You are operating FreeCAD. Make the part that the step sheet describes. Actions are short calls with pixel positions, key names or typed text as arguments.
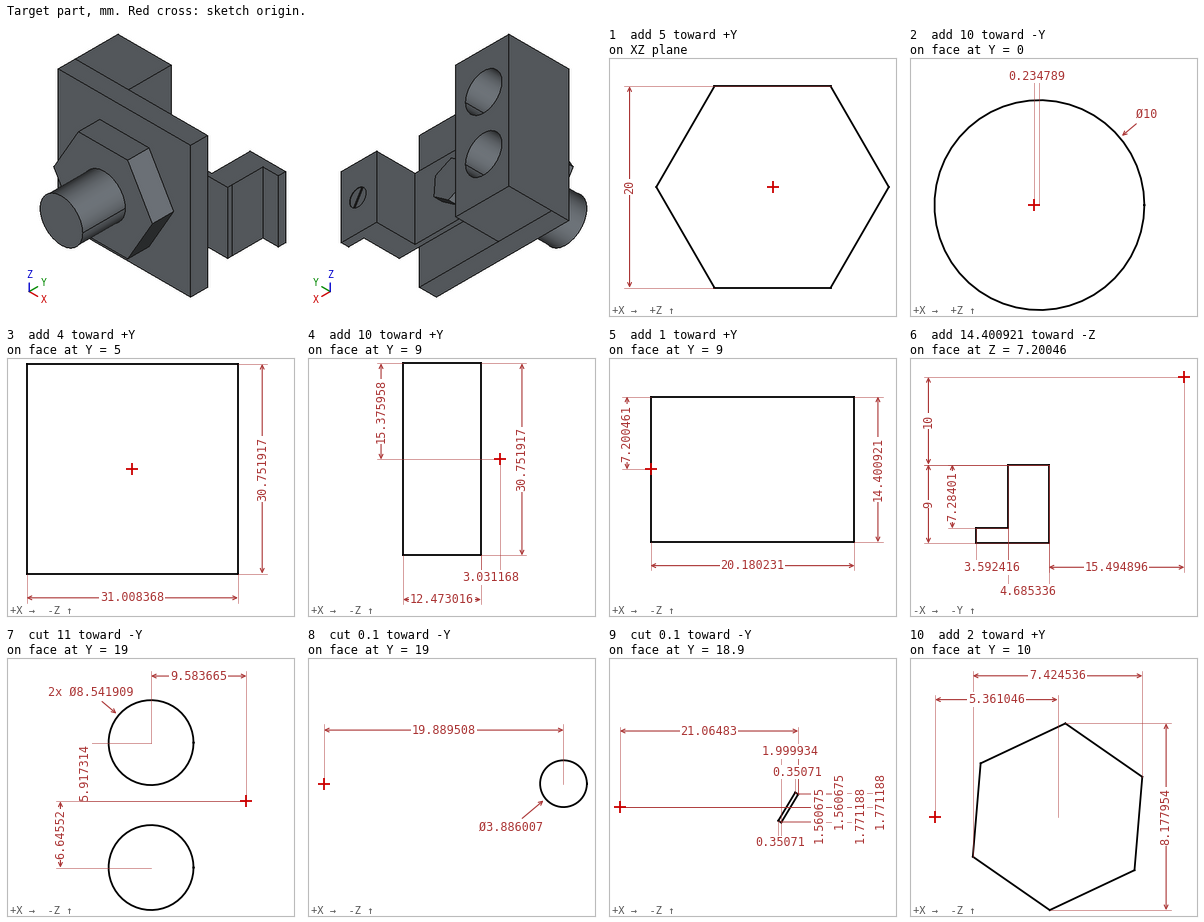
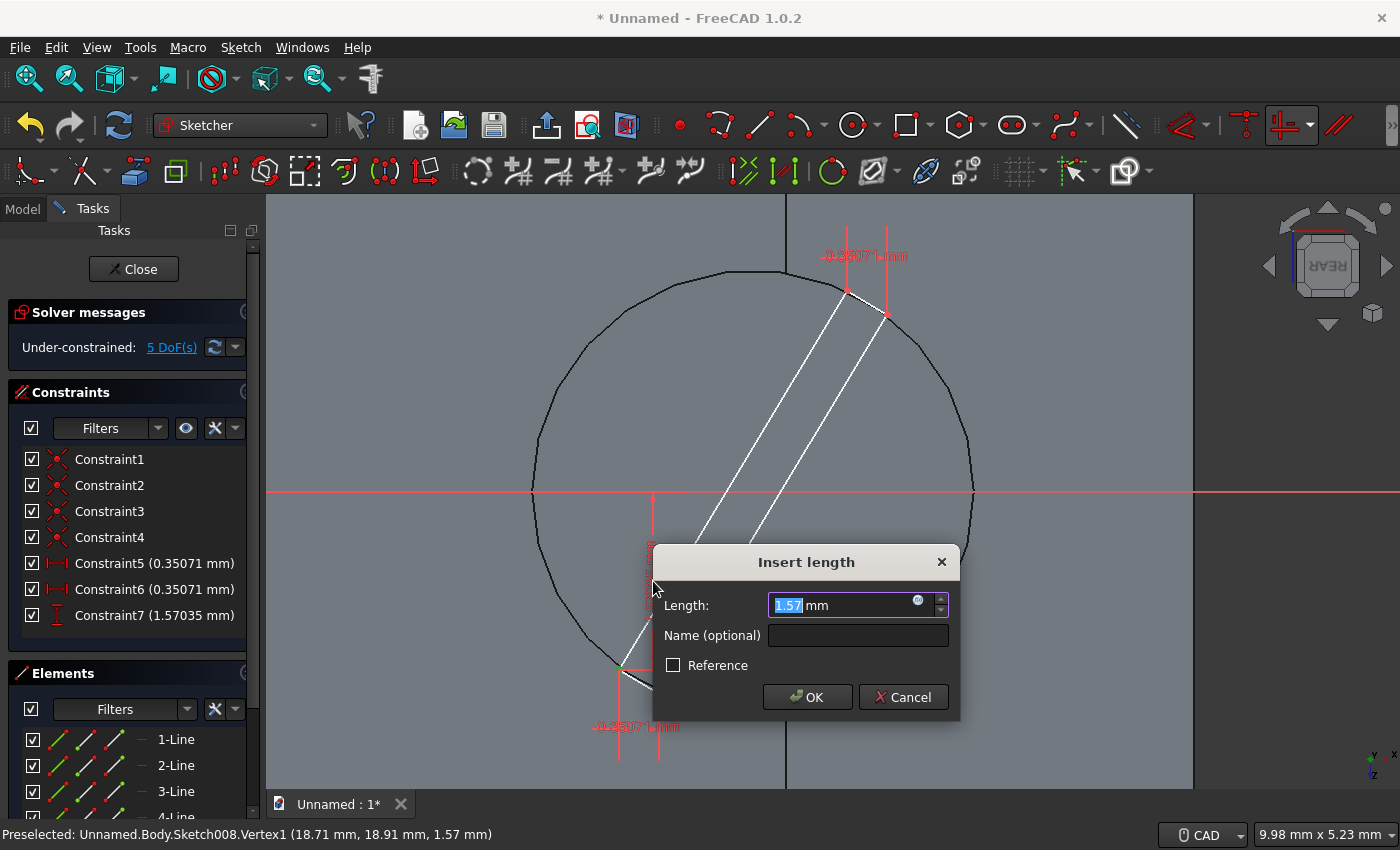
text(1.560675)
key(Return)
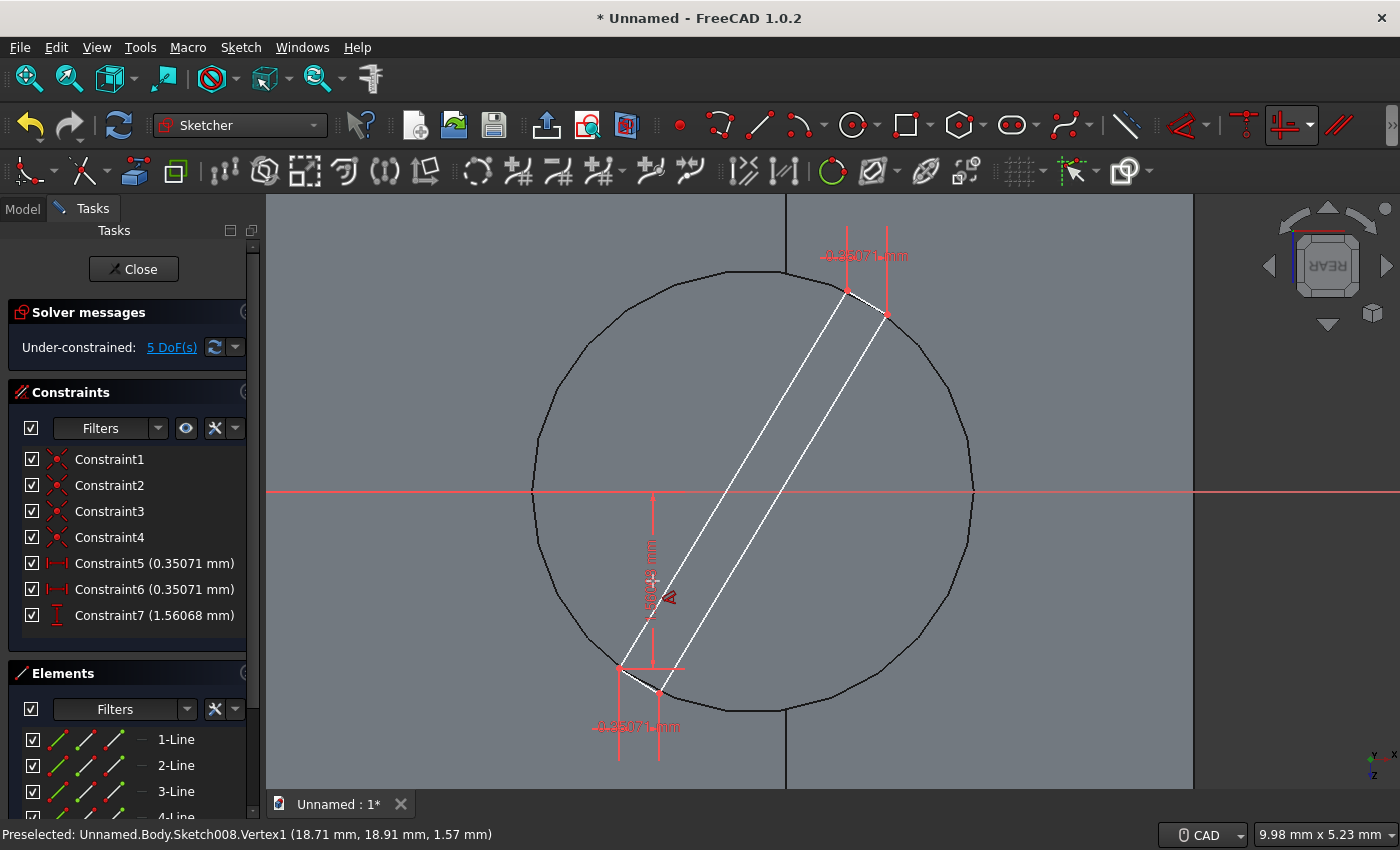
click(659, 694)
click(693, 664)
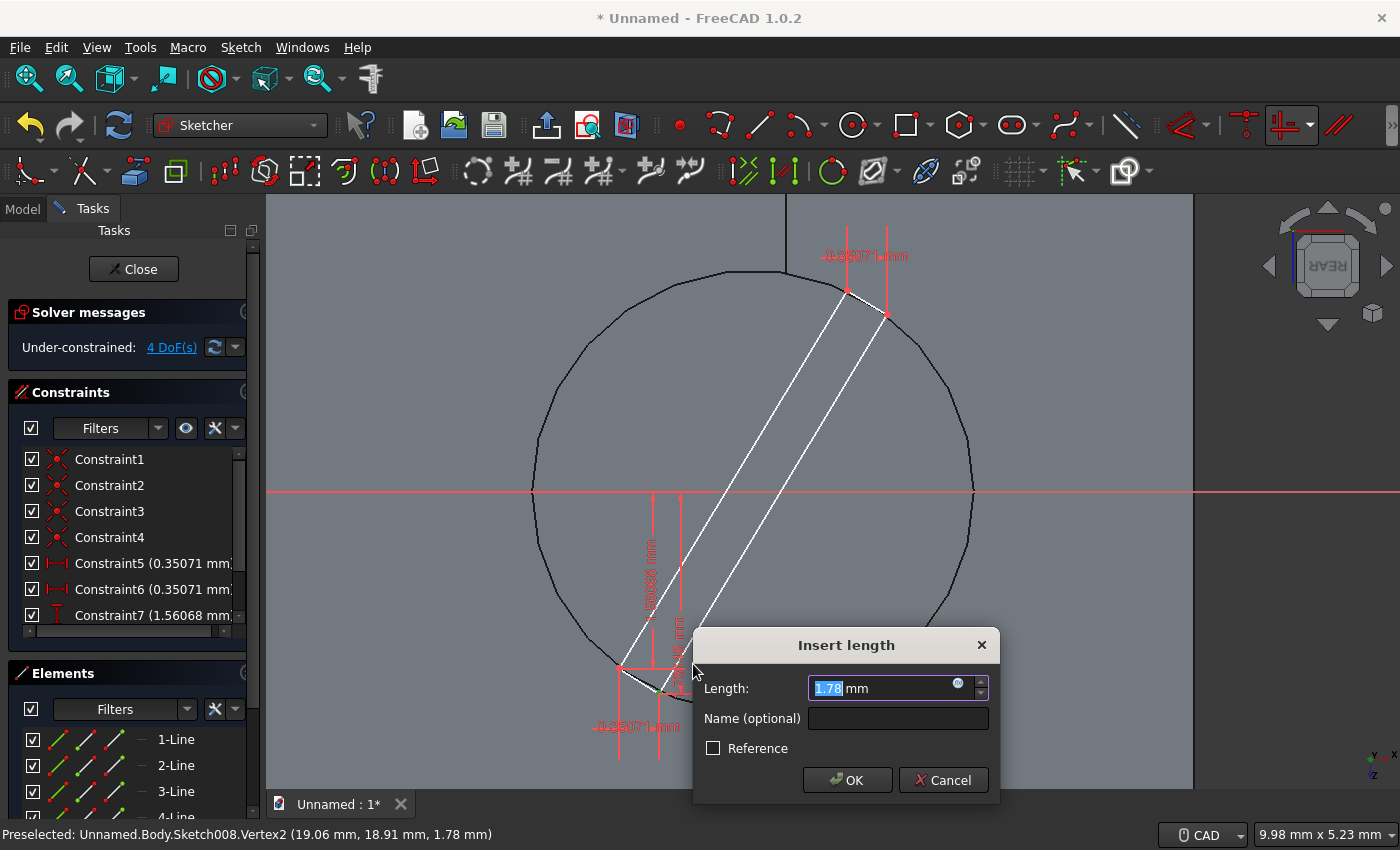
text(1.771188)
key(Return)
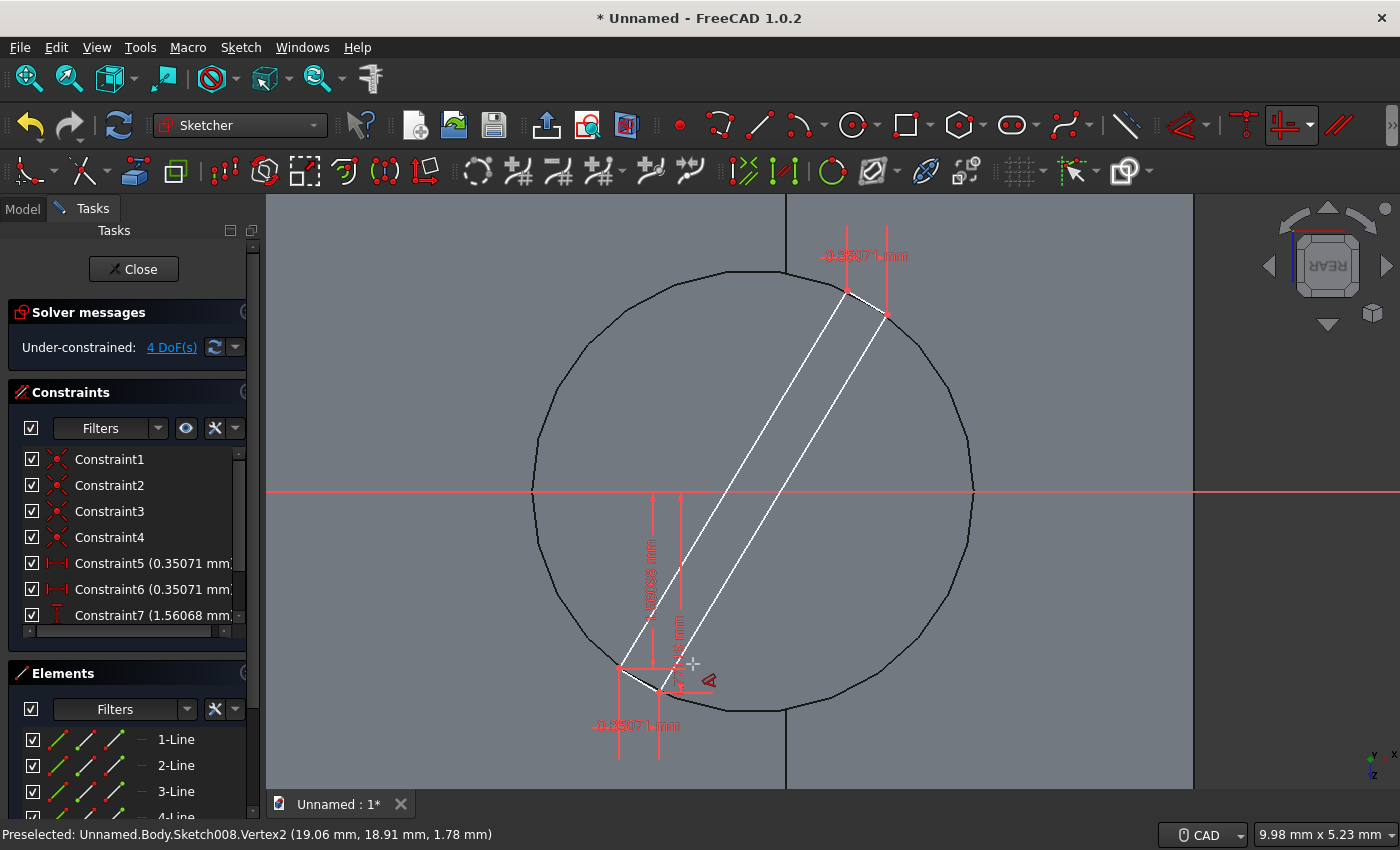
click(887, 315)
click(590, 281)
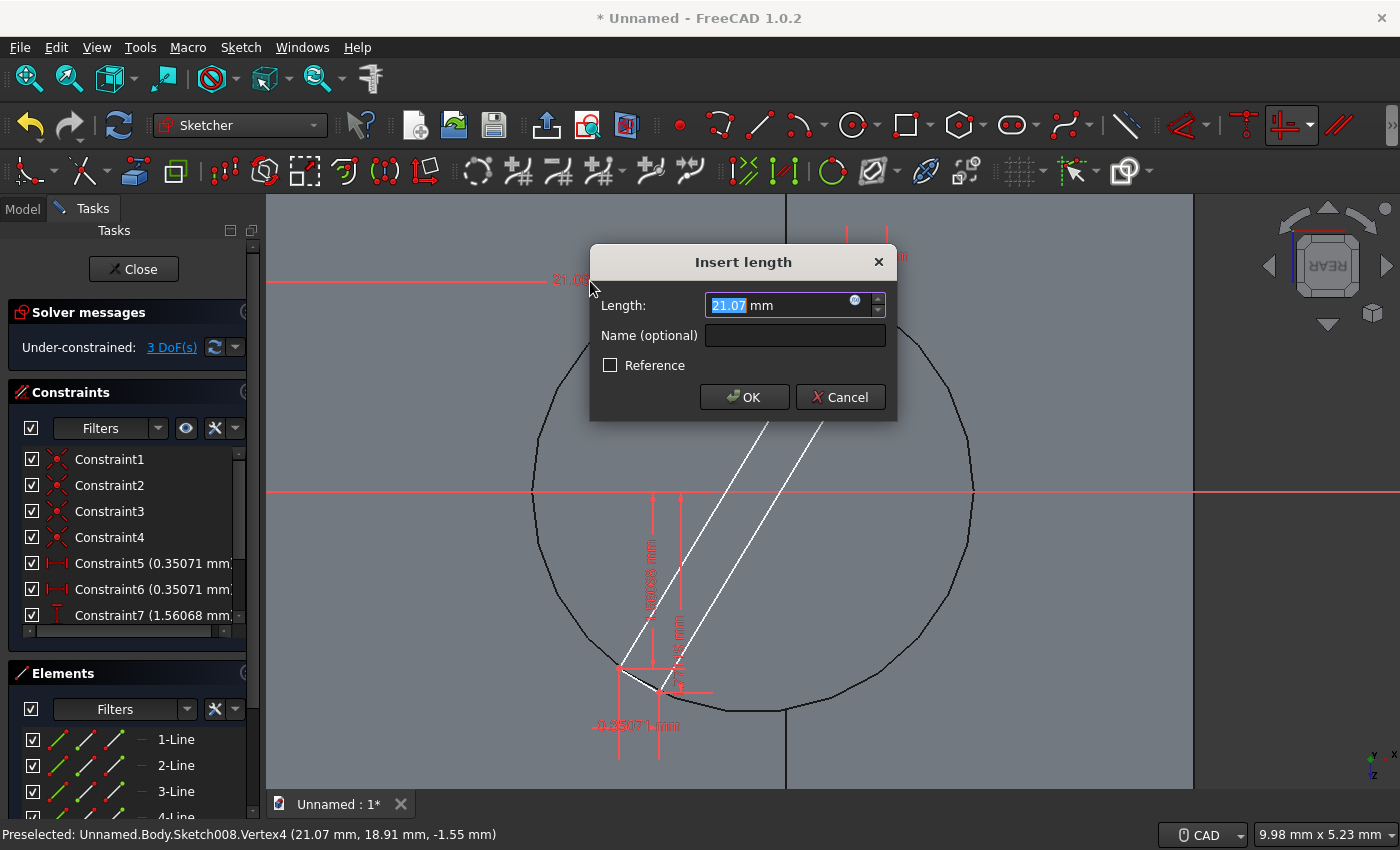
text(21.06483)
key(Return)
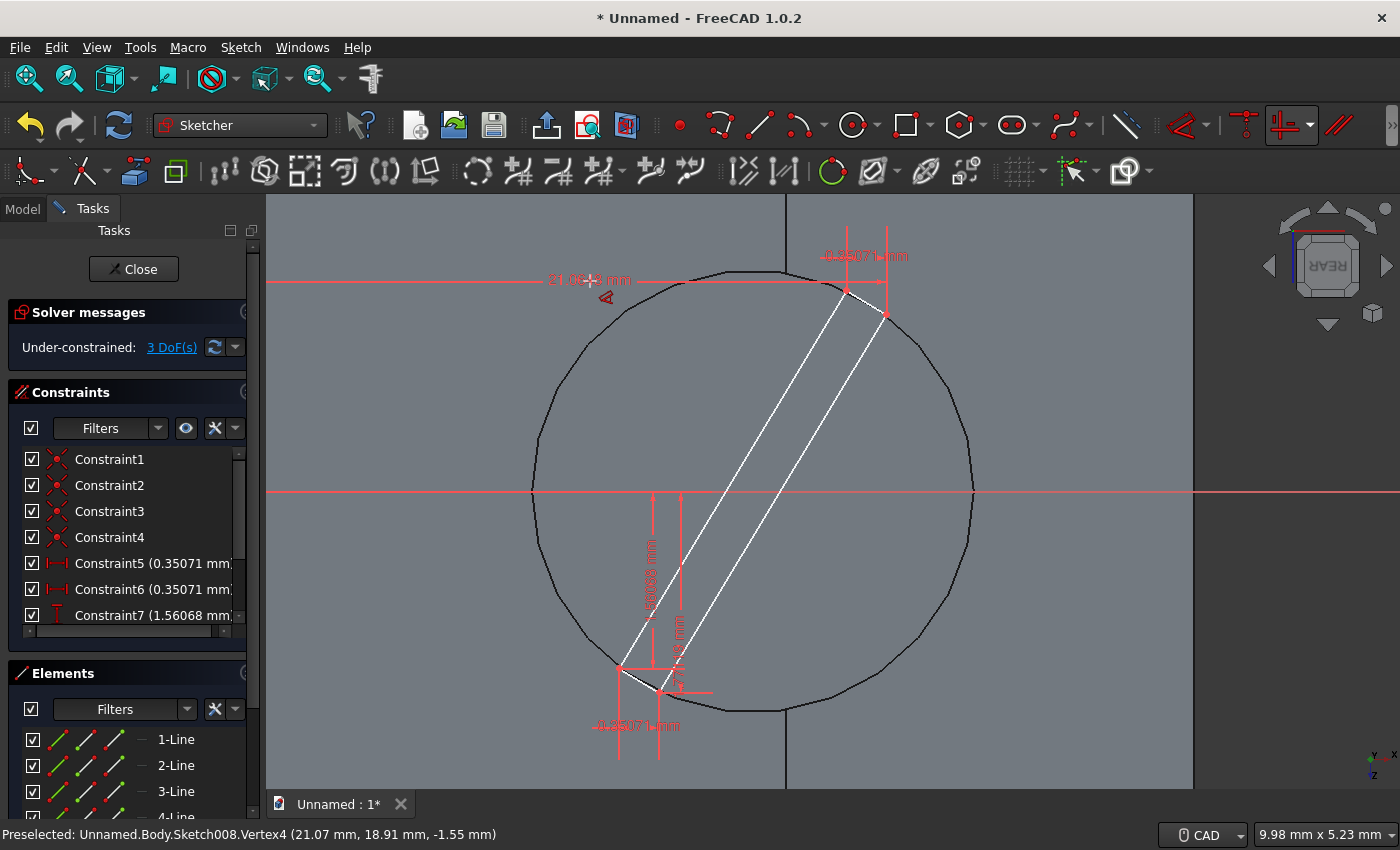
click(887, 315)
click(921, 403)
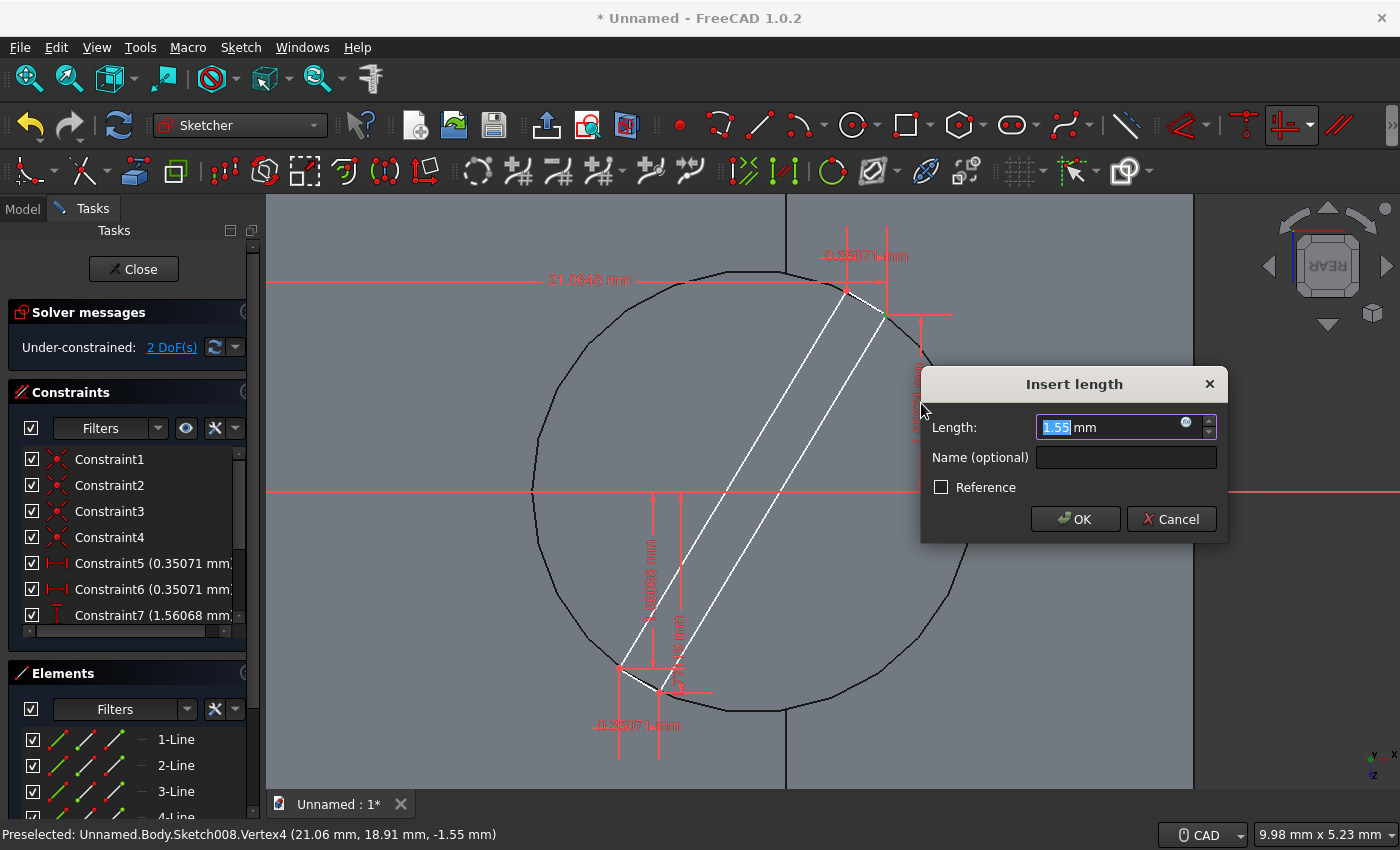
text(1.560675)
key(Return)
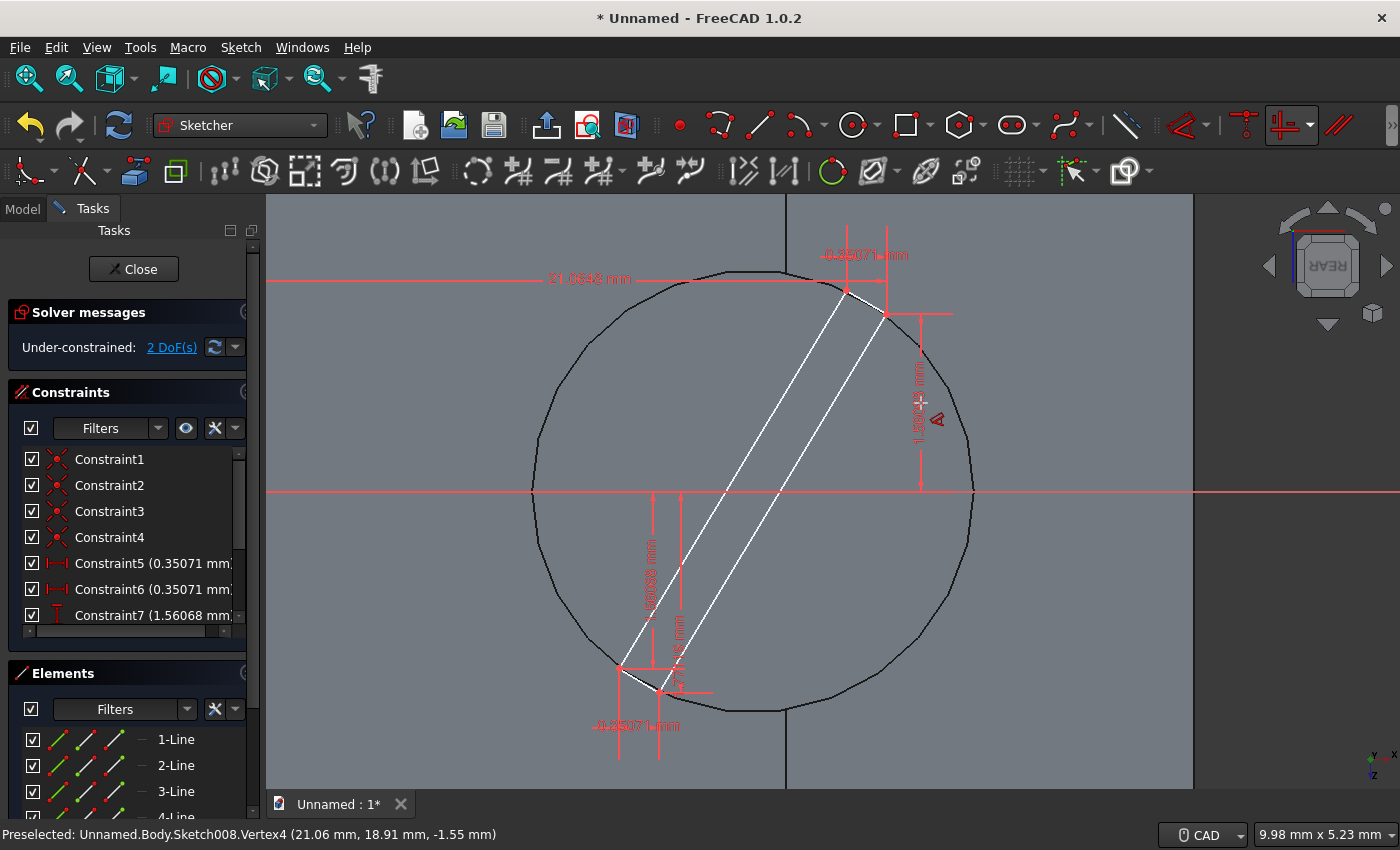
click(847, 291)
click(881, 437)